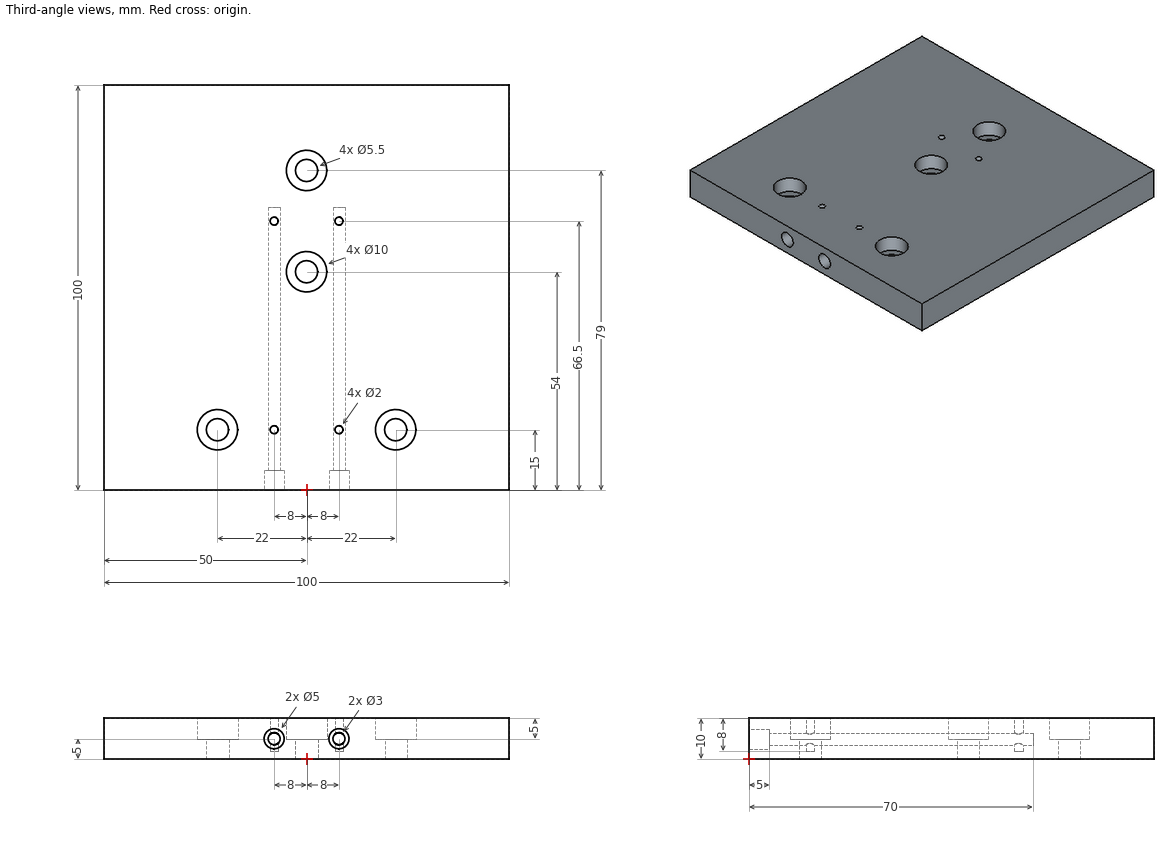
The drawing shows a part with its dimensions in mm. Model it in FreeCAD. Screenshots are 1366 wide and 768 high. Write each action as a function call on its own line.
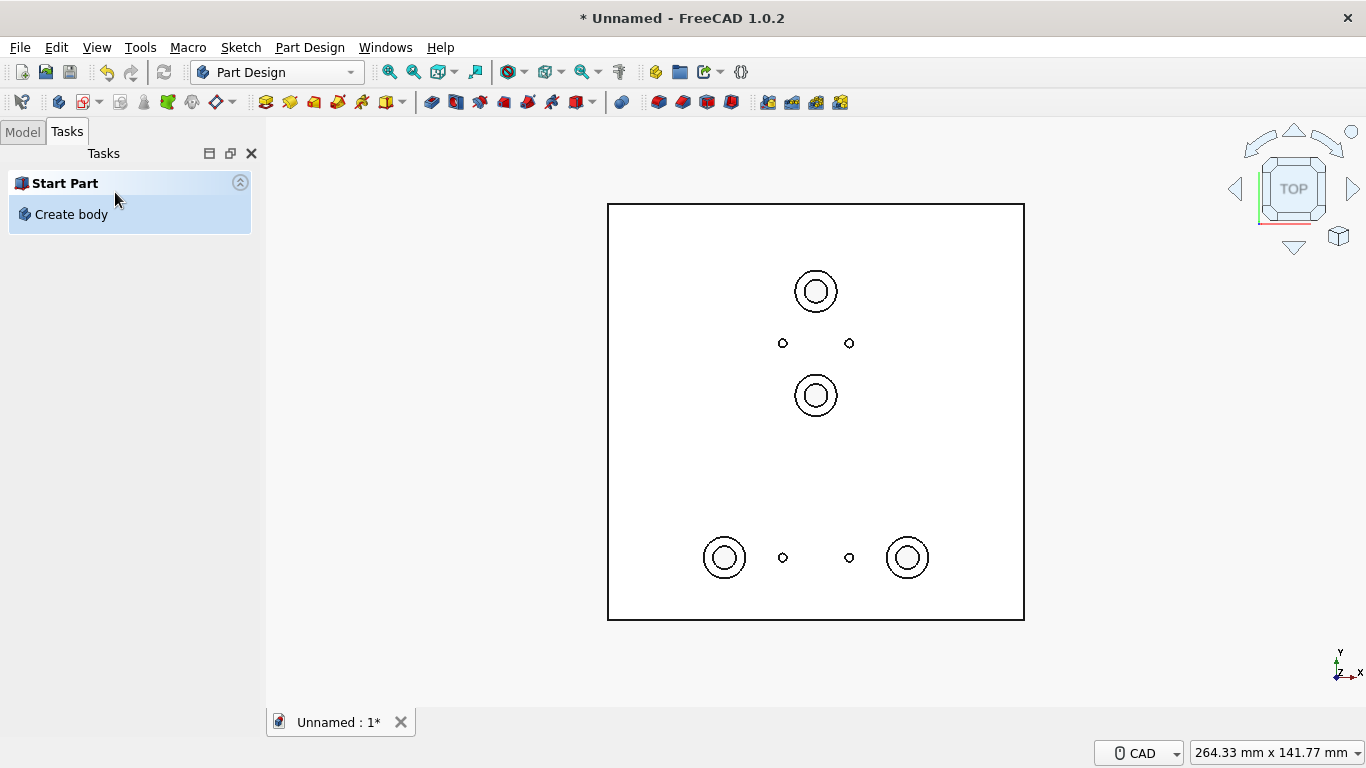
key(0)